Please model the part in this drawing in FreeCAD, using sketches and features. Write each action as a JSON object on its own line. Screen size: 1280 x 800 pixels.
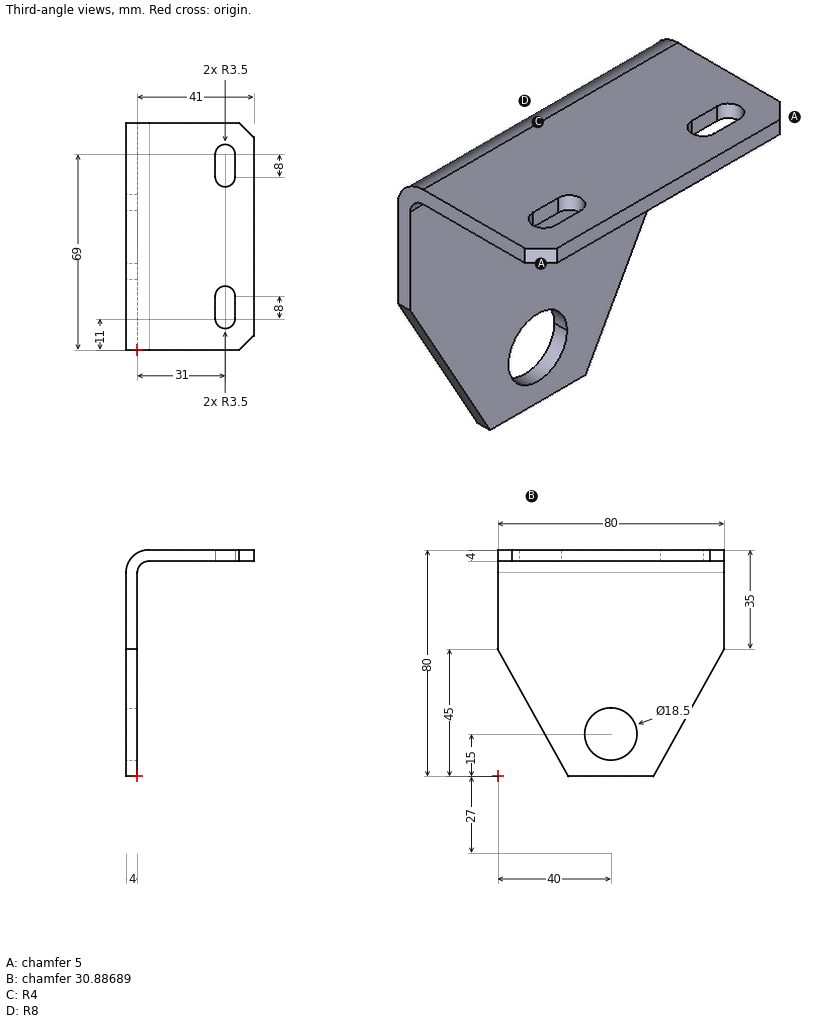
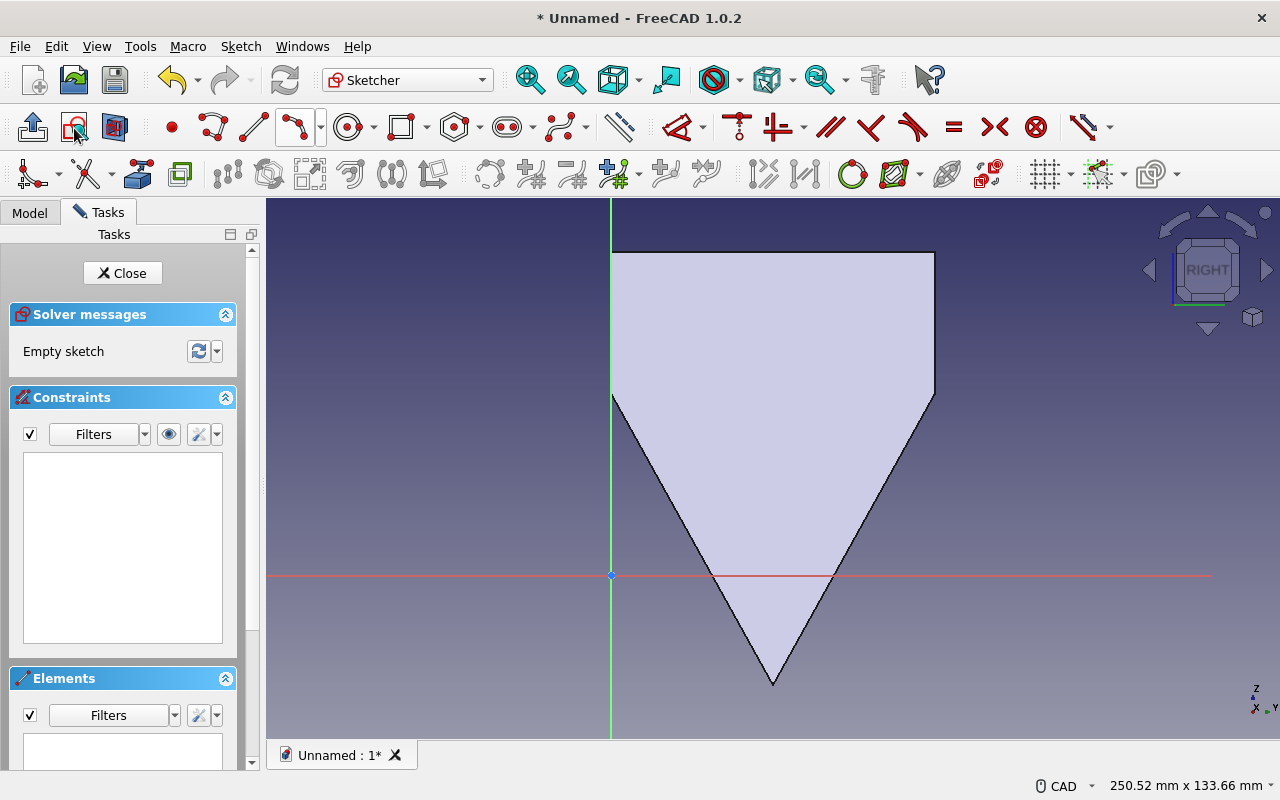
{"action": "key", "text": "g r"}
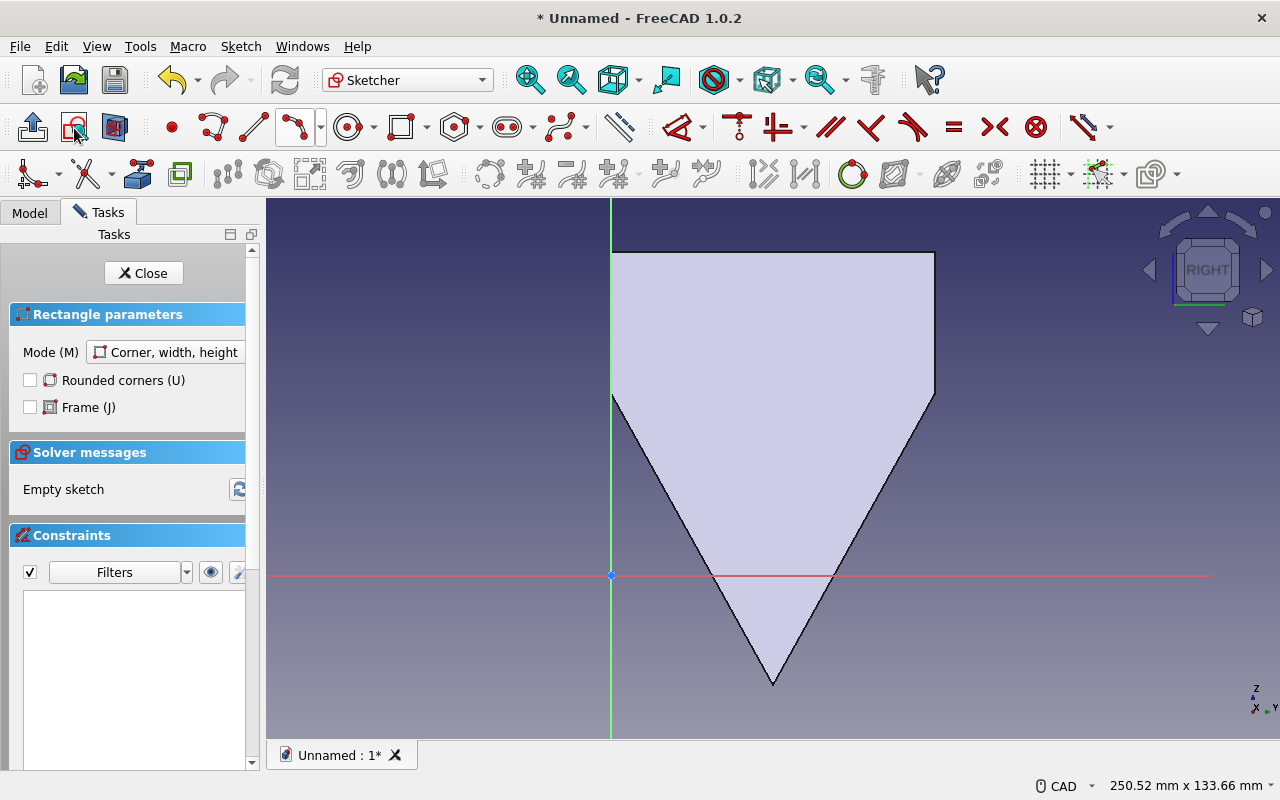
{"action": "left_click", "coordinate": [611, 252]}
{"action": "left_click", "coordinate": [935, 268]}
{"action": "key", "text": "Escape"}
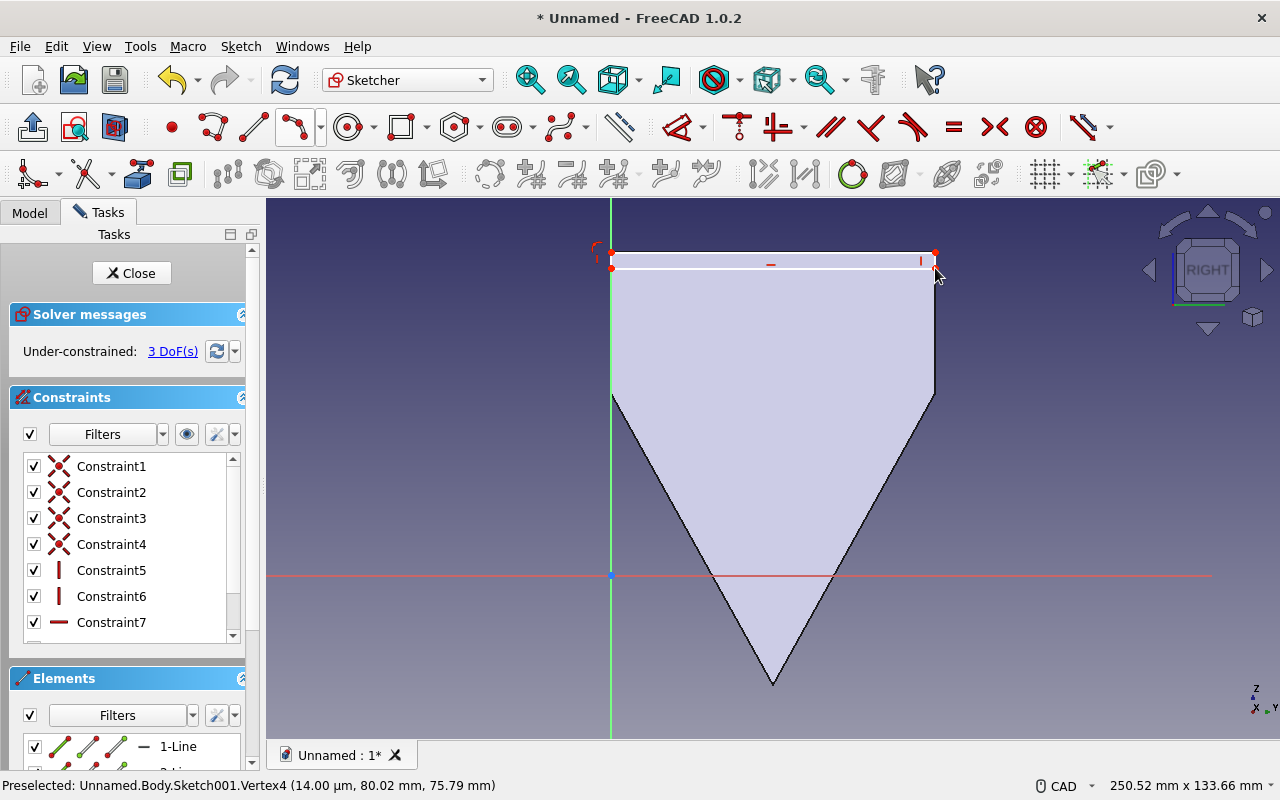
{"action": "left_click", "coordinate": [676, 128]}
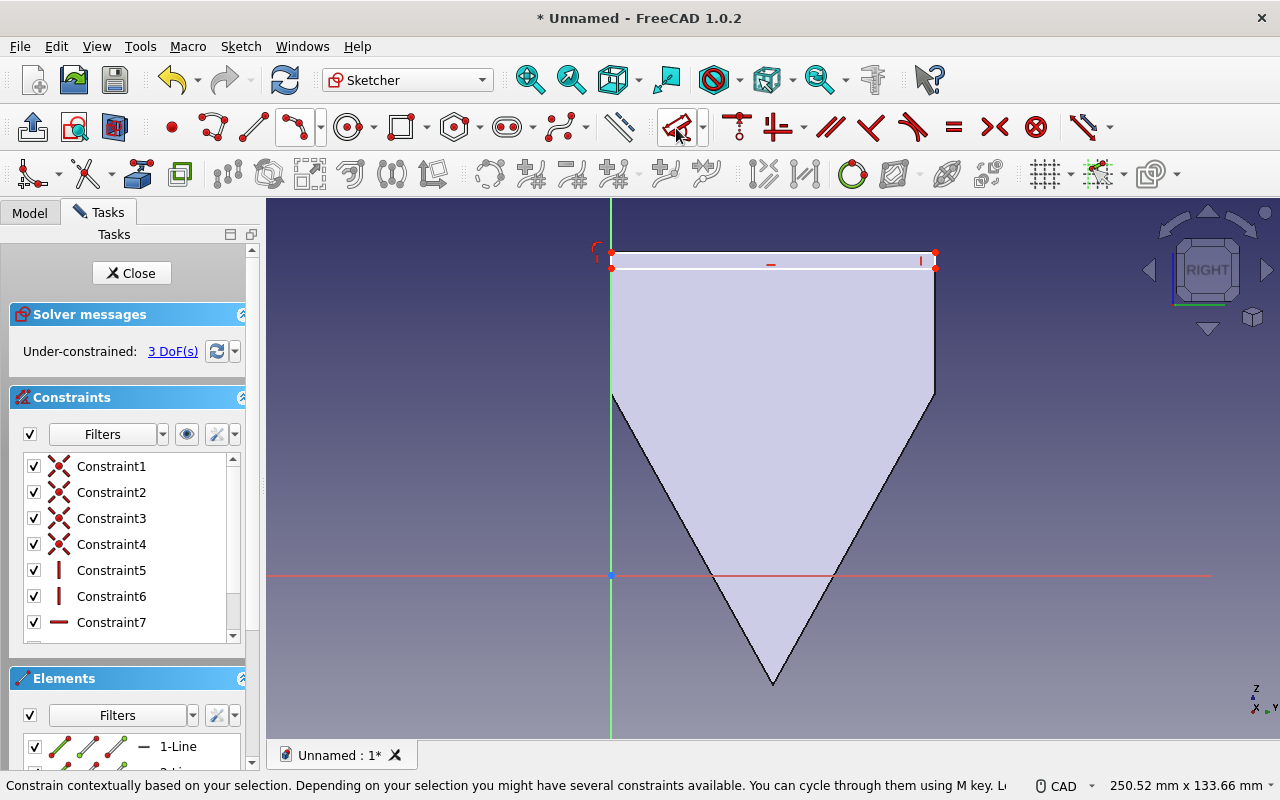
{"action": "scroll", "coordinate": [611, 261], "scroll_direction": "up", "scroll_amount": 5}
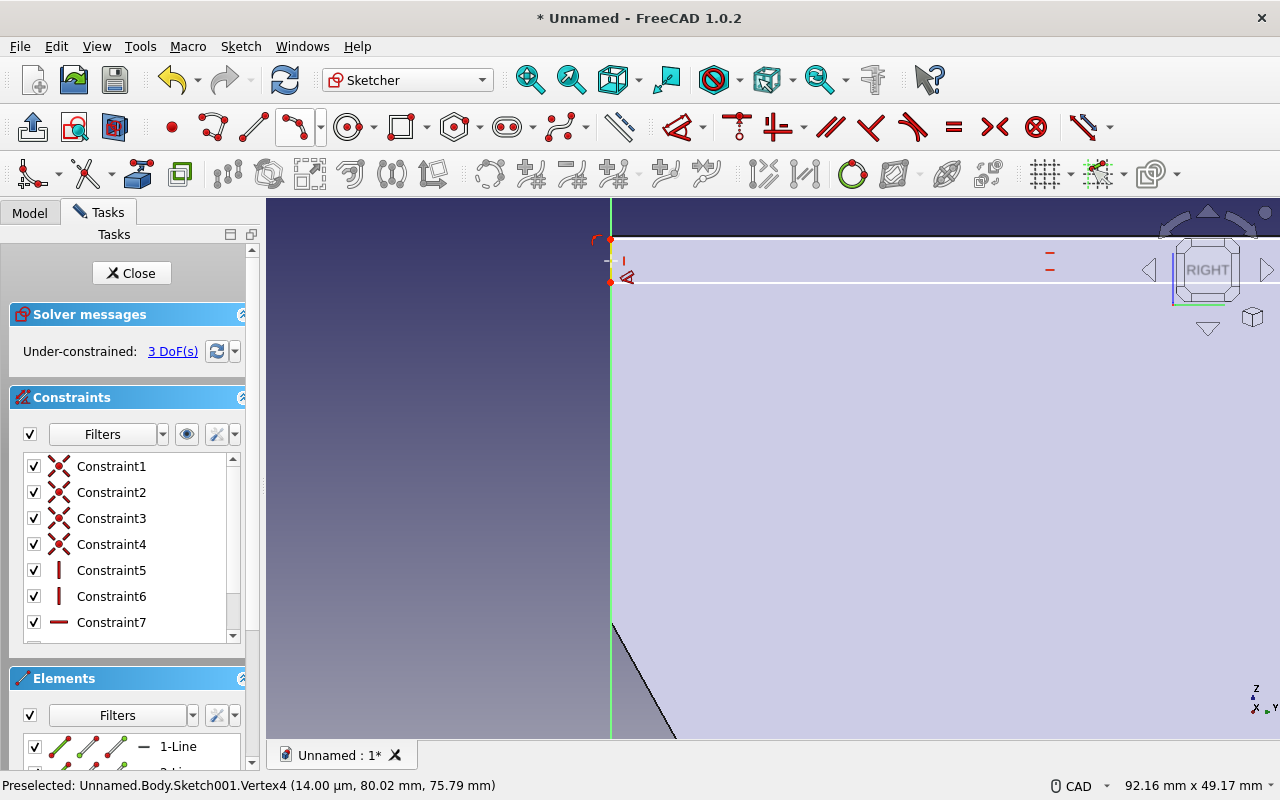
{"action": "left_click", "coordinate": [611, 261]}
{"action": "left_click", "coordinate": [577, 261]}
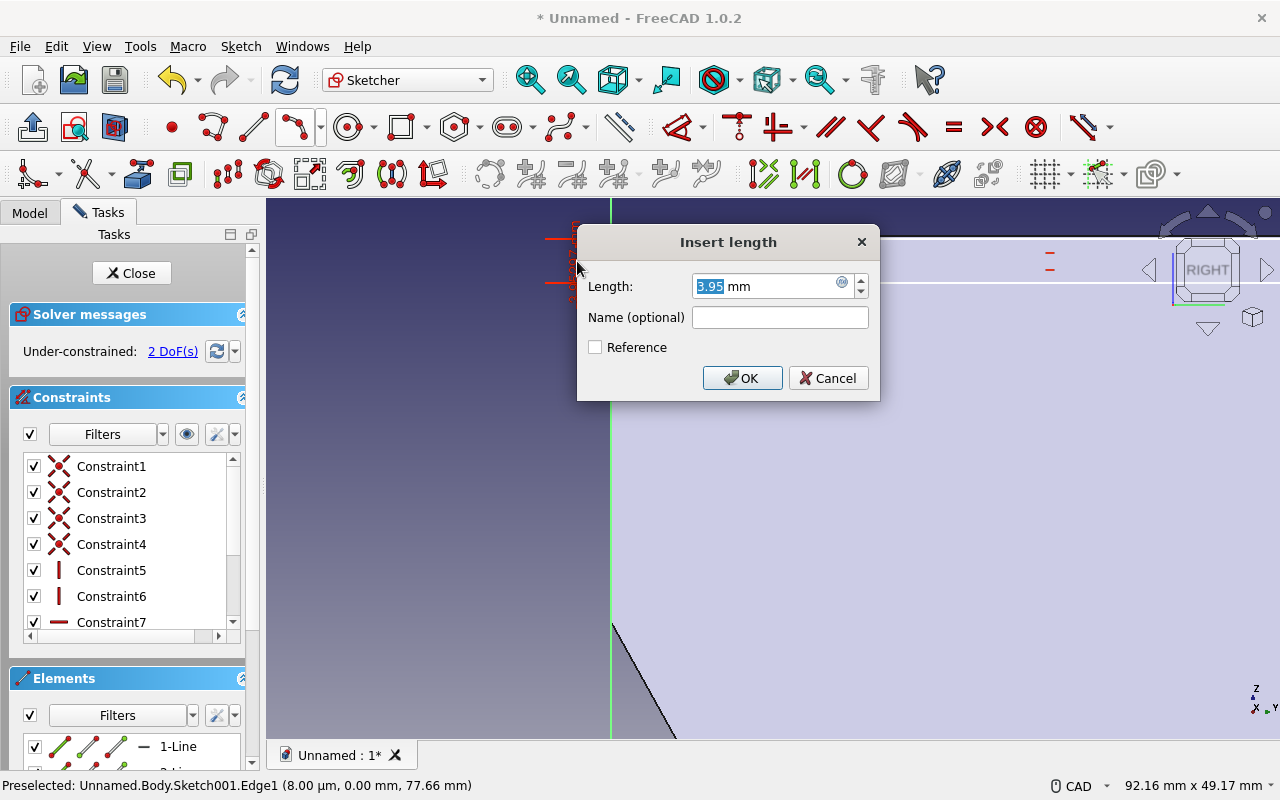
{"action": "type", "text": "4"}
{"action": "key", "text": "Return"}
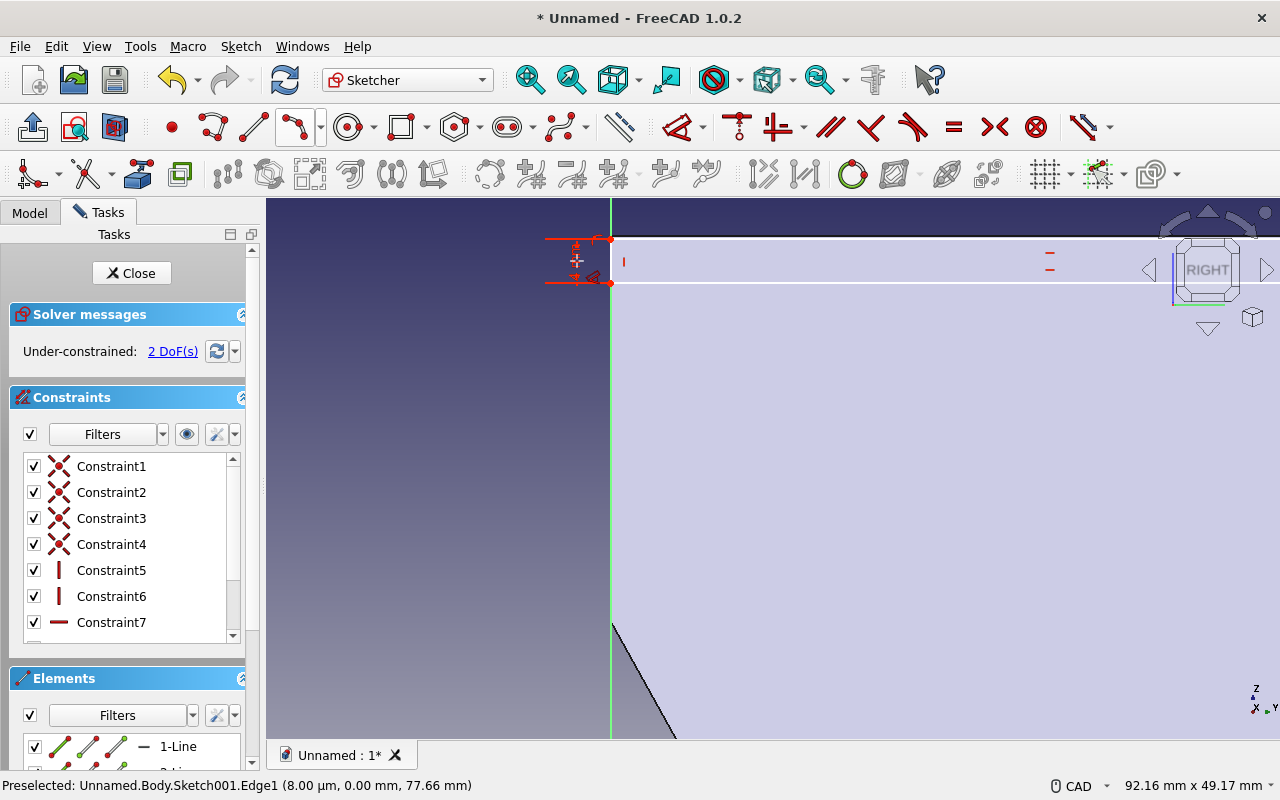
{"action": "left_click", "coordinate": [875, 283]}
{"action": "left_click", "coordinate": [863, 317]}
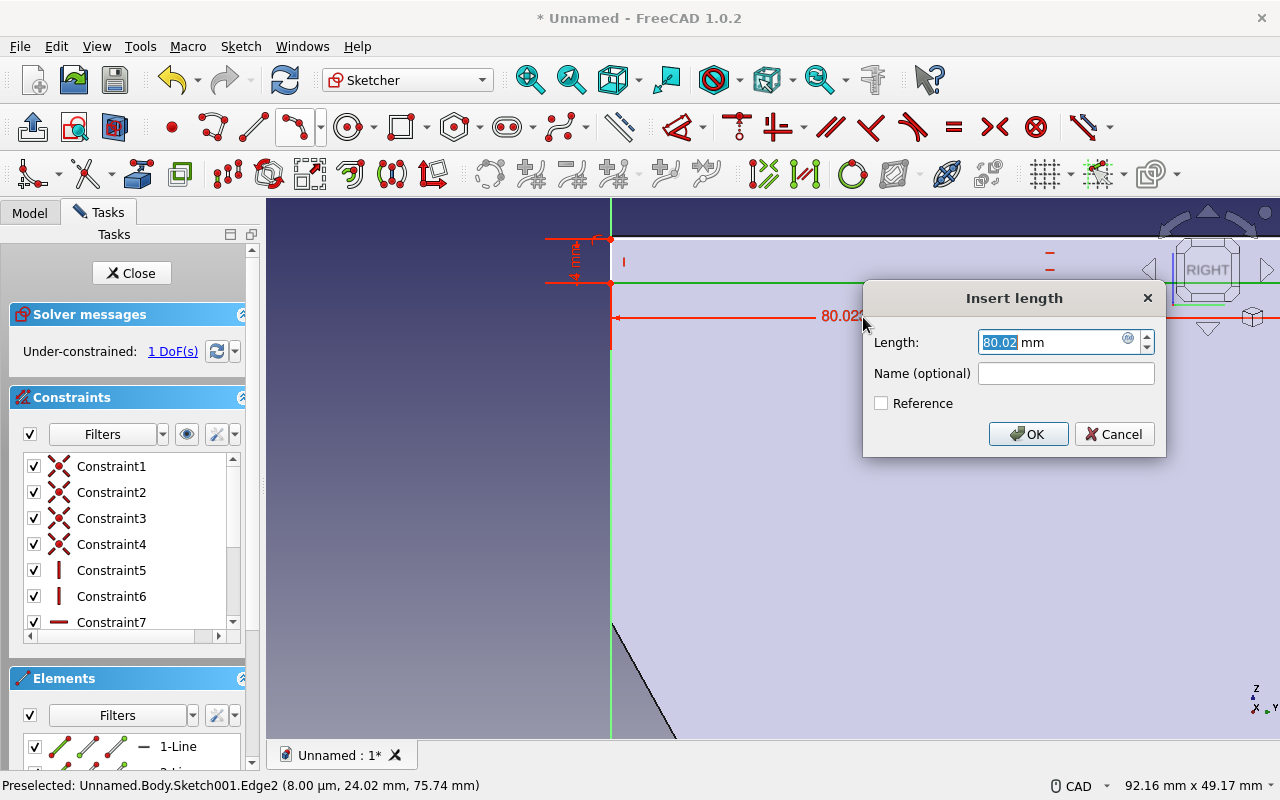
{"action": "type", "text": "80"}
{"action": "key", "text": "Return"}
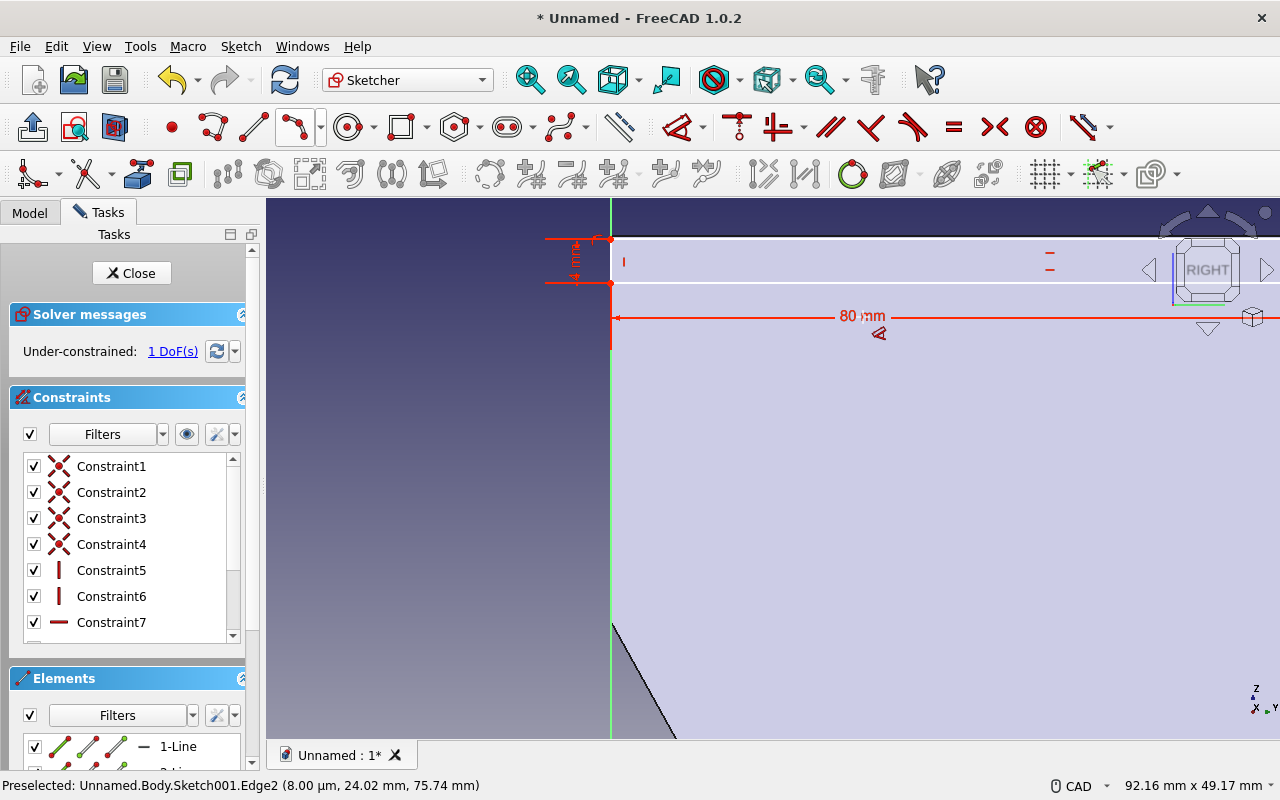
{"action": "left_click", "coordinate": [611, 239]}
{"action": "left_click", "coordinate": [577, 475]}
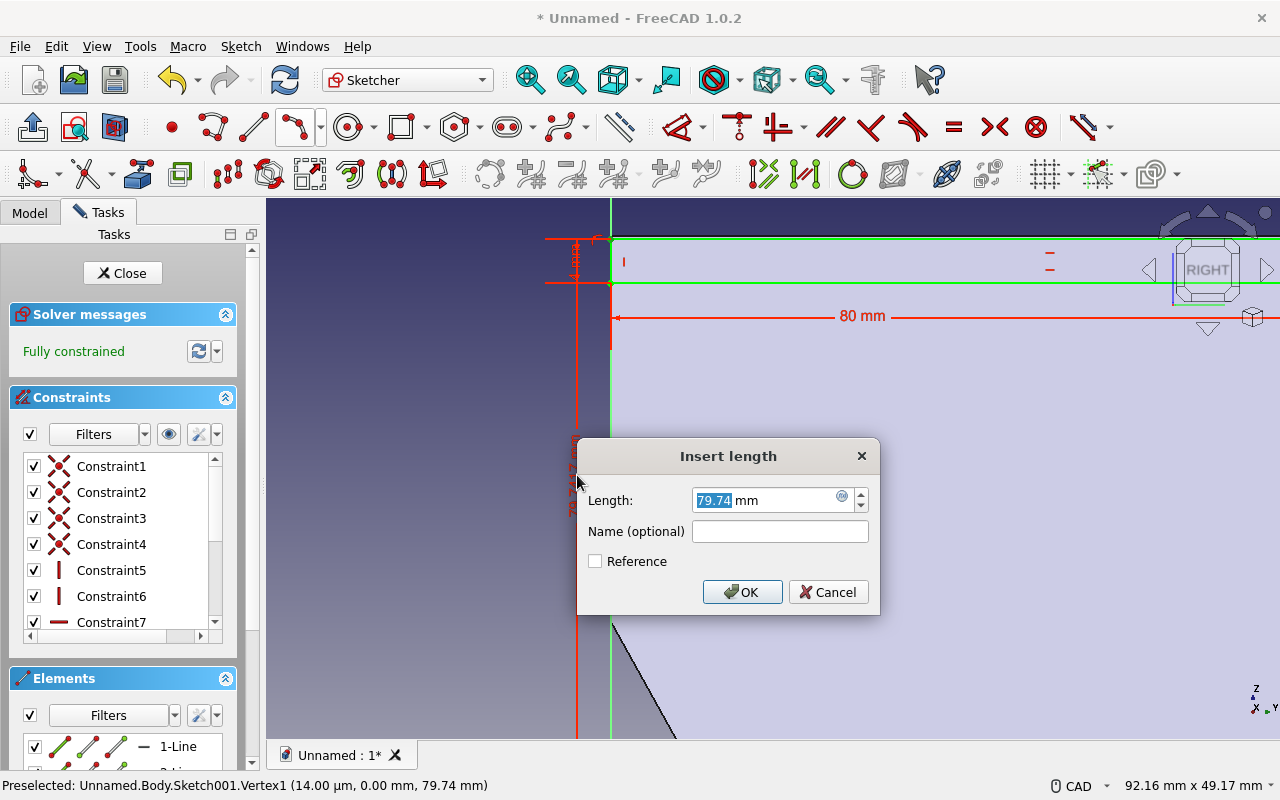
{"action": "type", "text": "80"}
{"action": "key", "text": "Return"}
{"action": "key", "text": "Escape"}